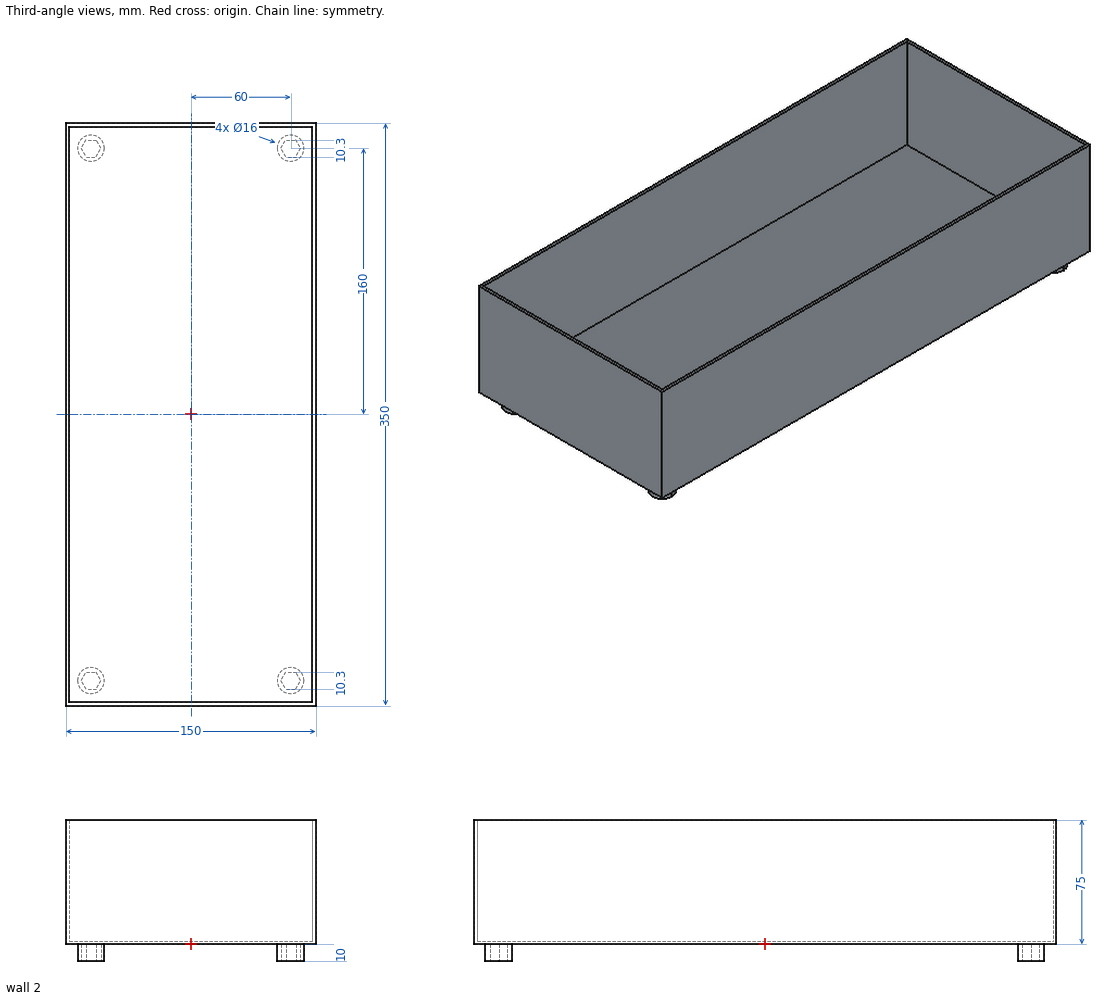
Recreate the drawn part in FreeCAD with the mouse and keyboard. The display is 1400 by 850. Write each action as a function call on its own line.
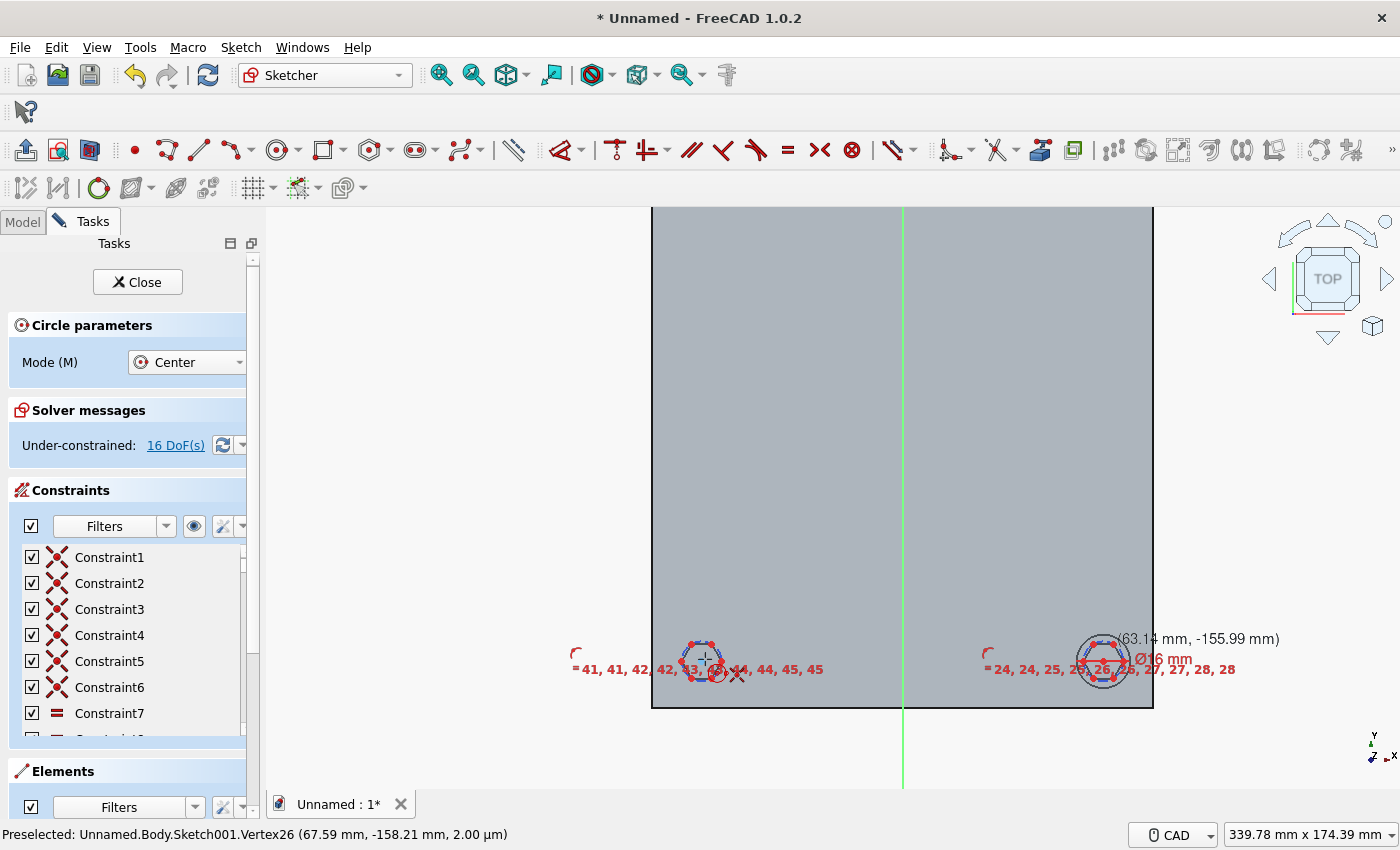
click(702, 661)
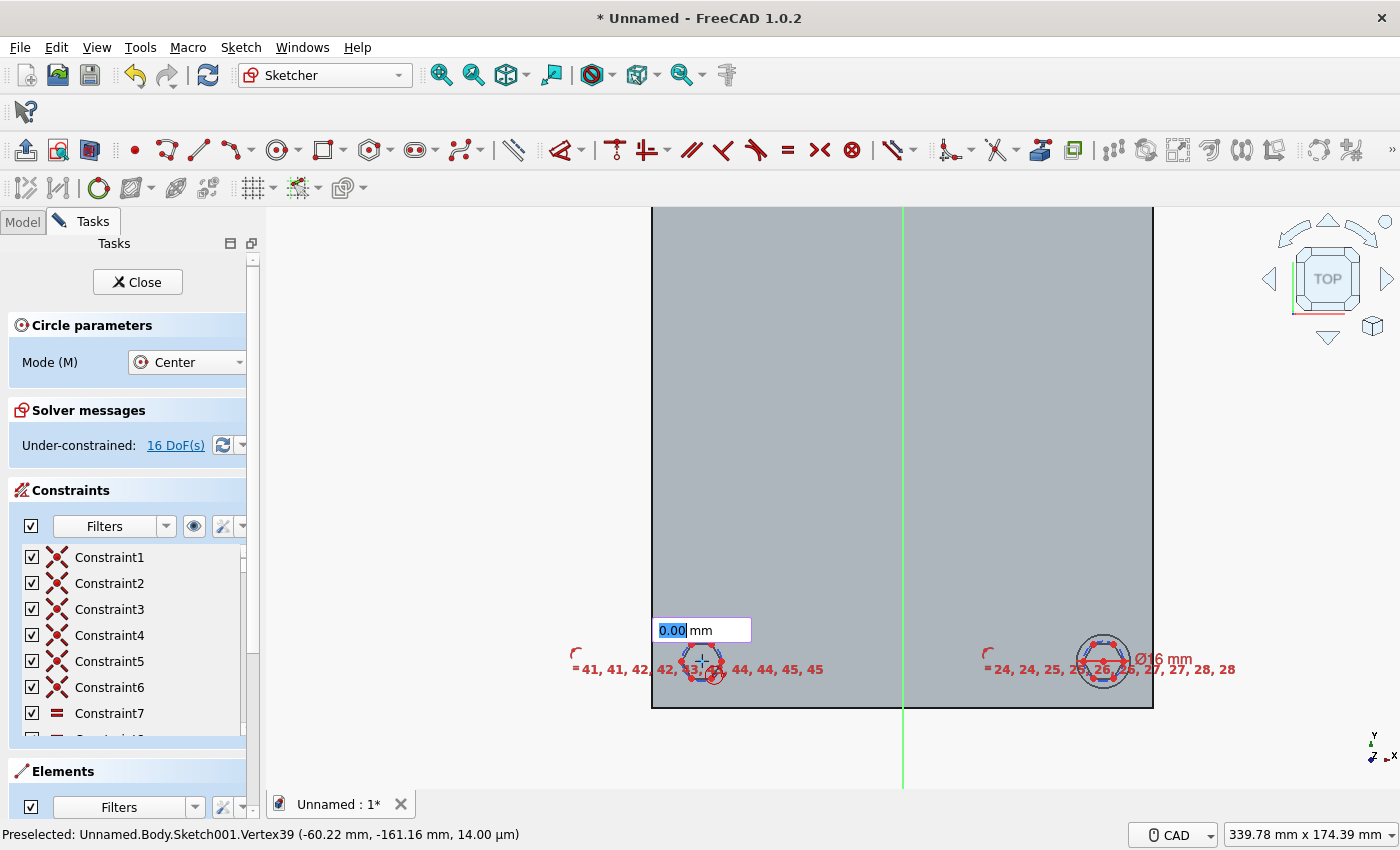
scroll(728, 648, up, 3)
move(727, 648)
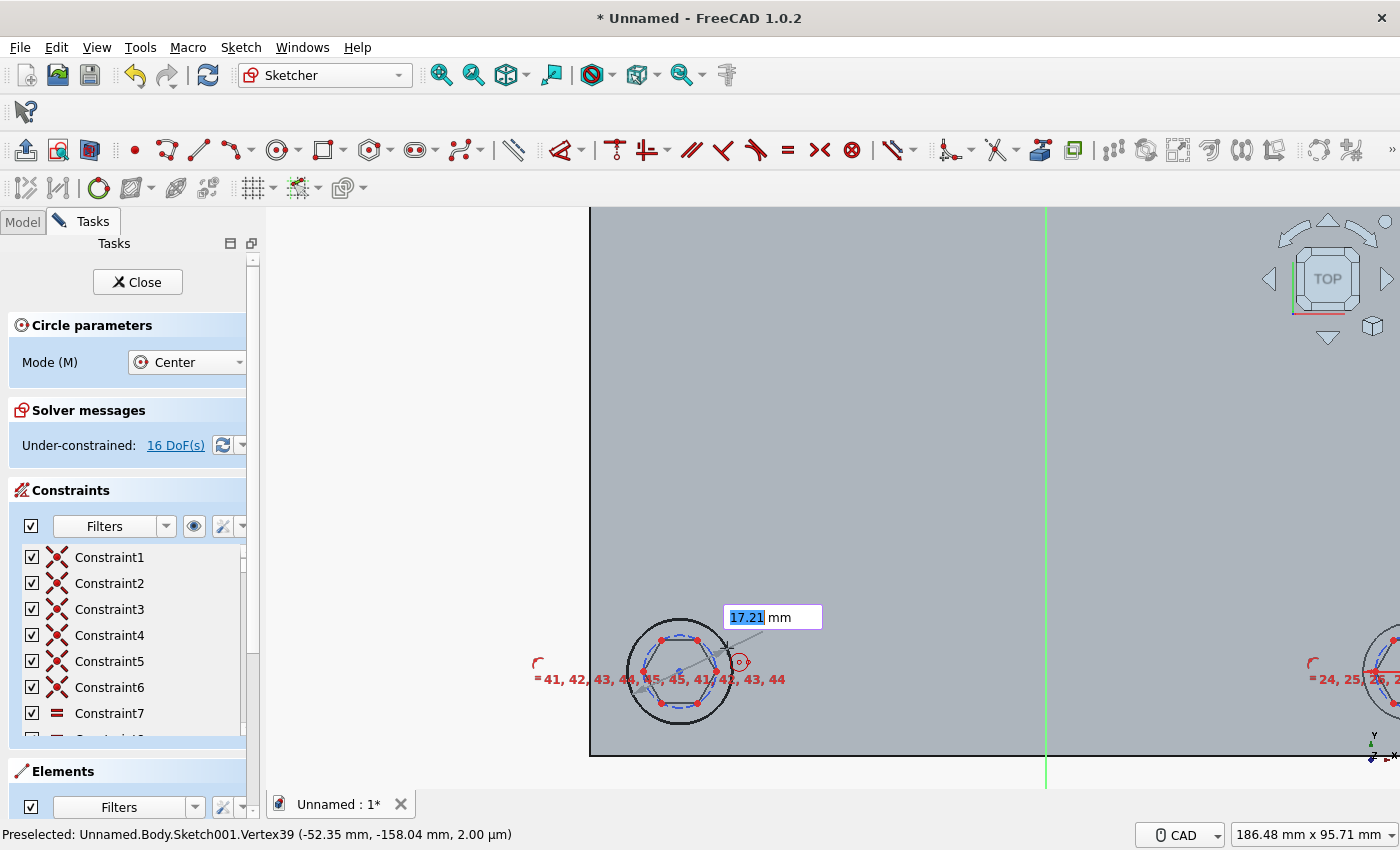
text(16)
key(Return)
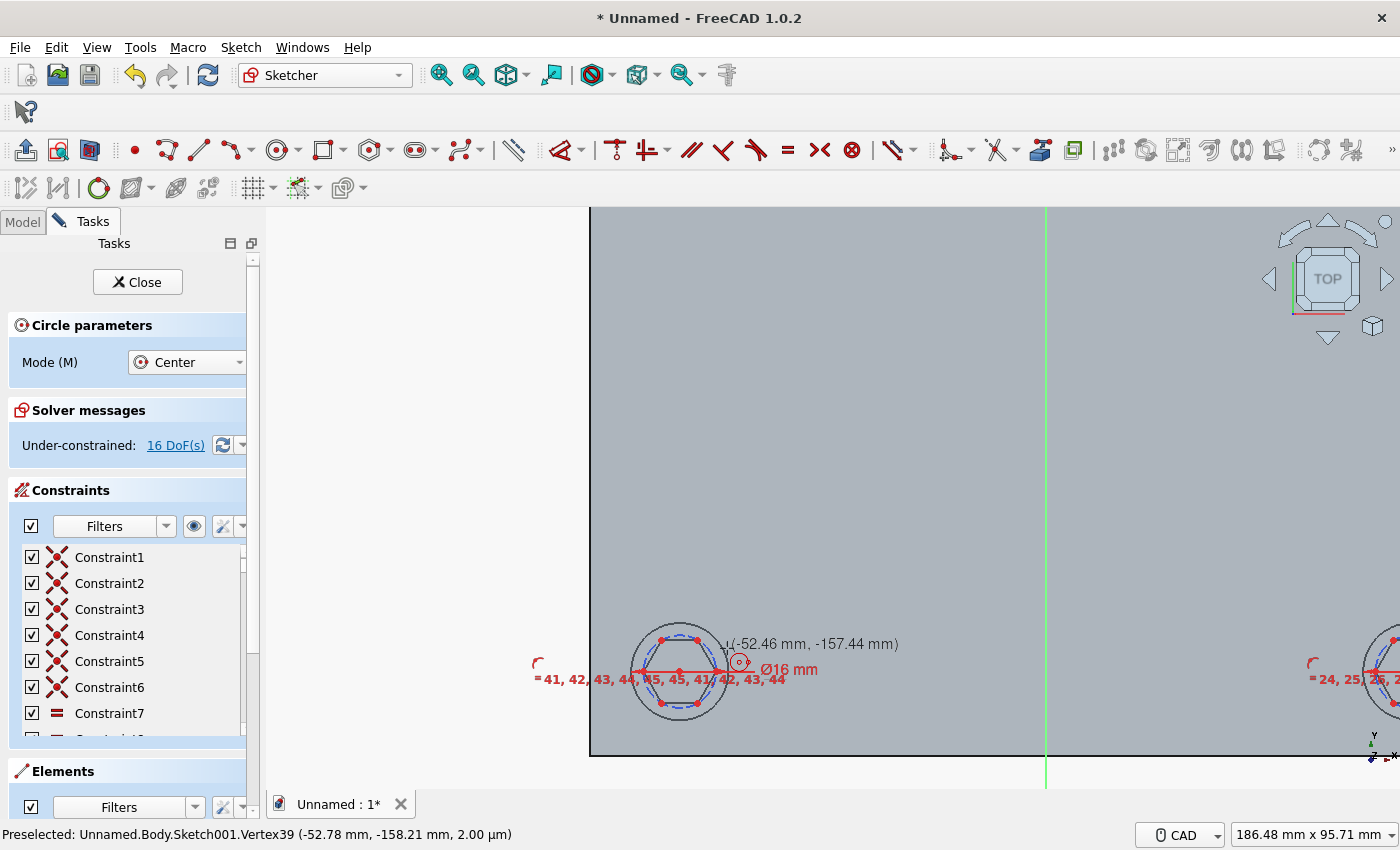
scroll(709, 658, down, 9)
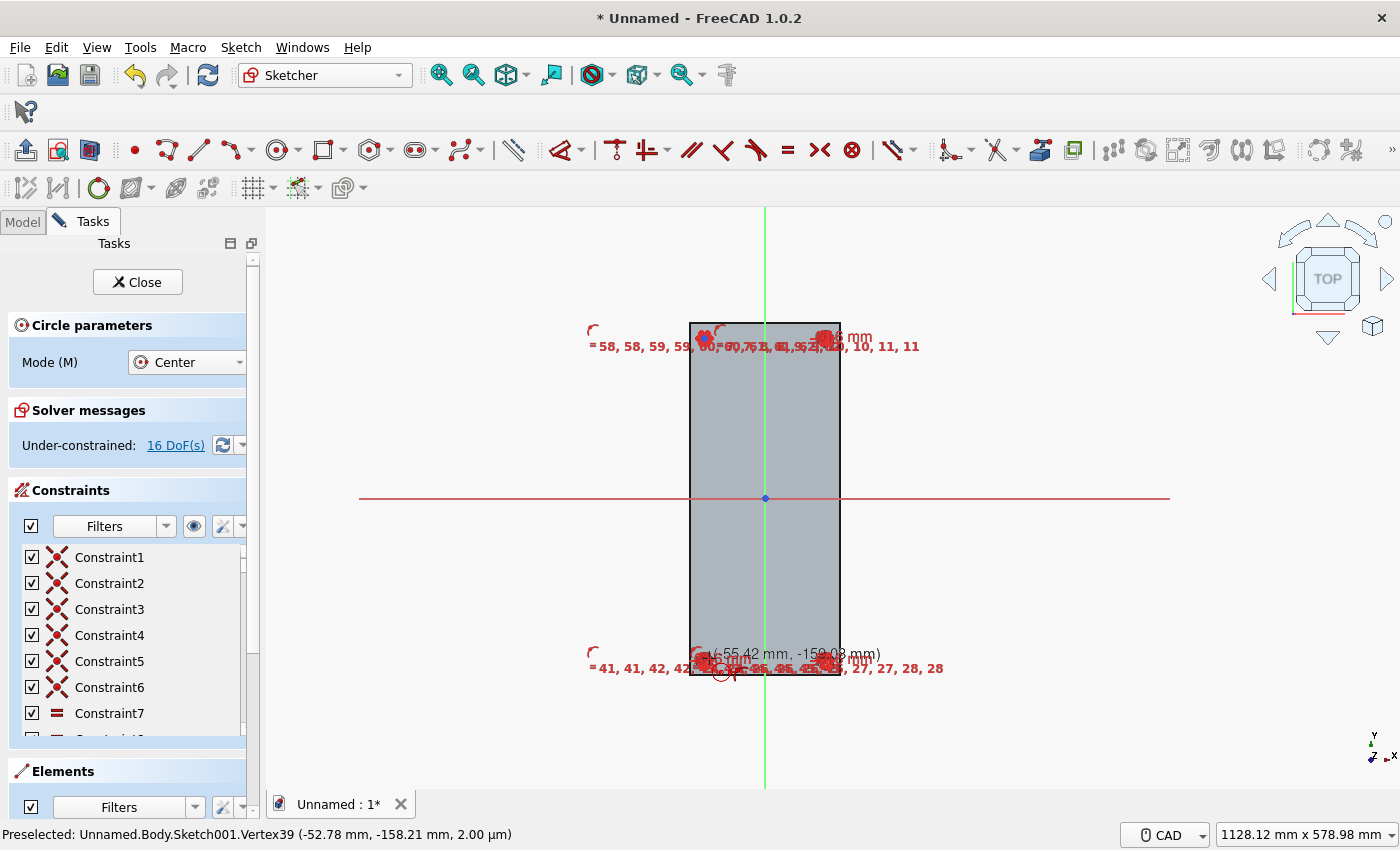
scroll(705, 338, up, 6)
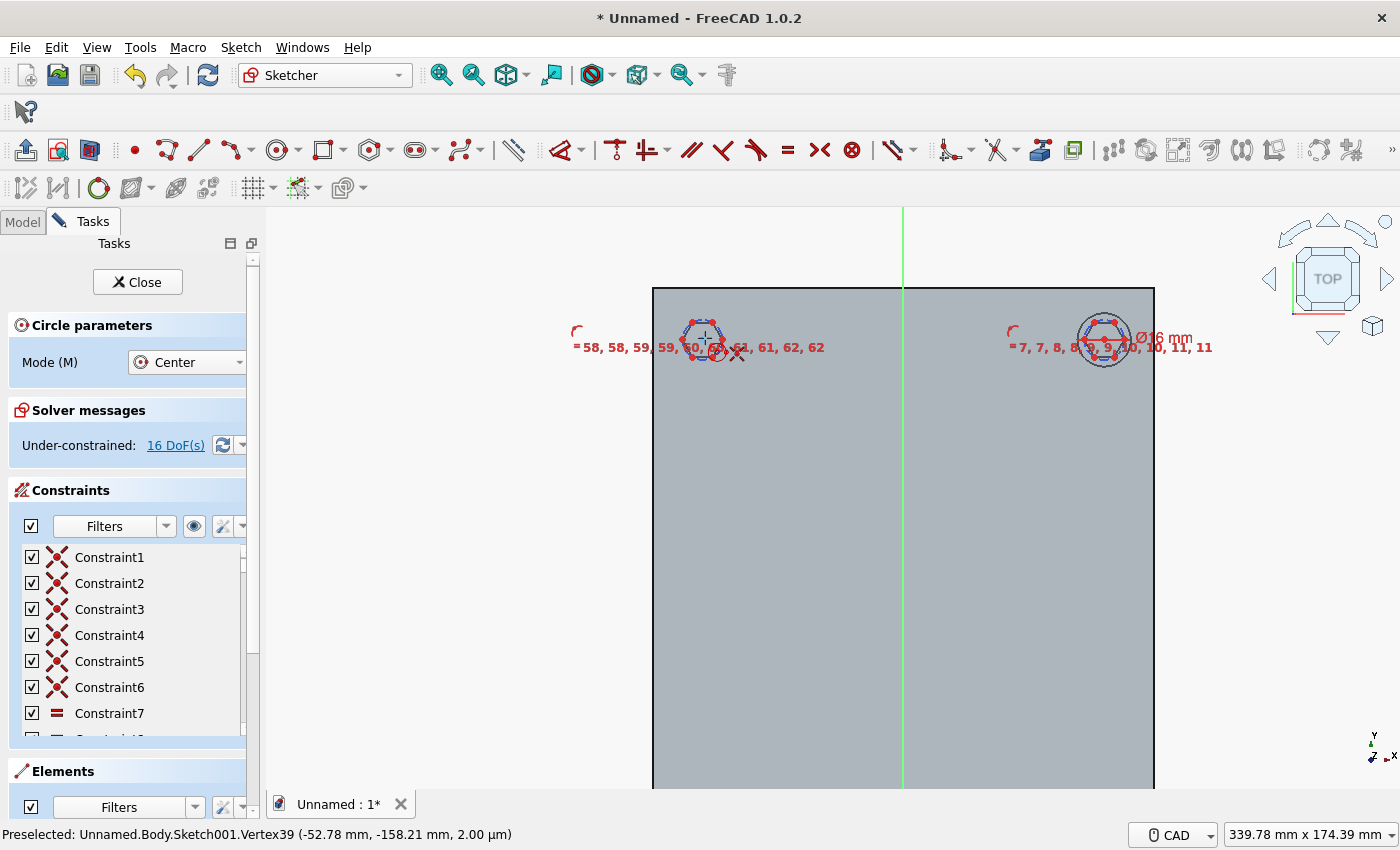
click(702, 340)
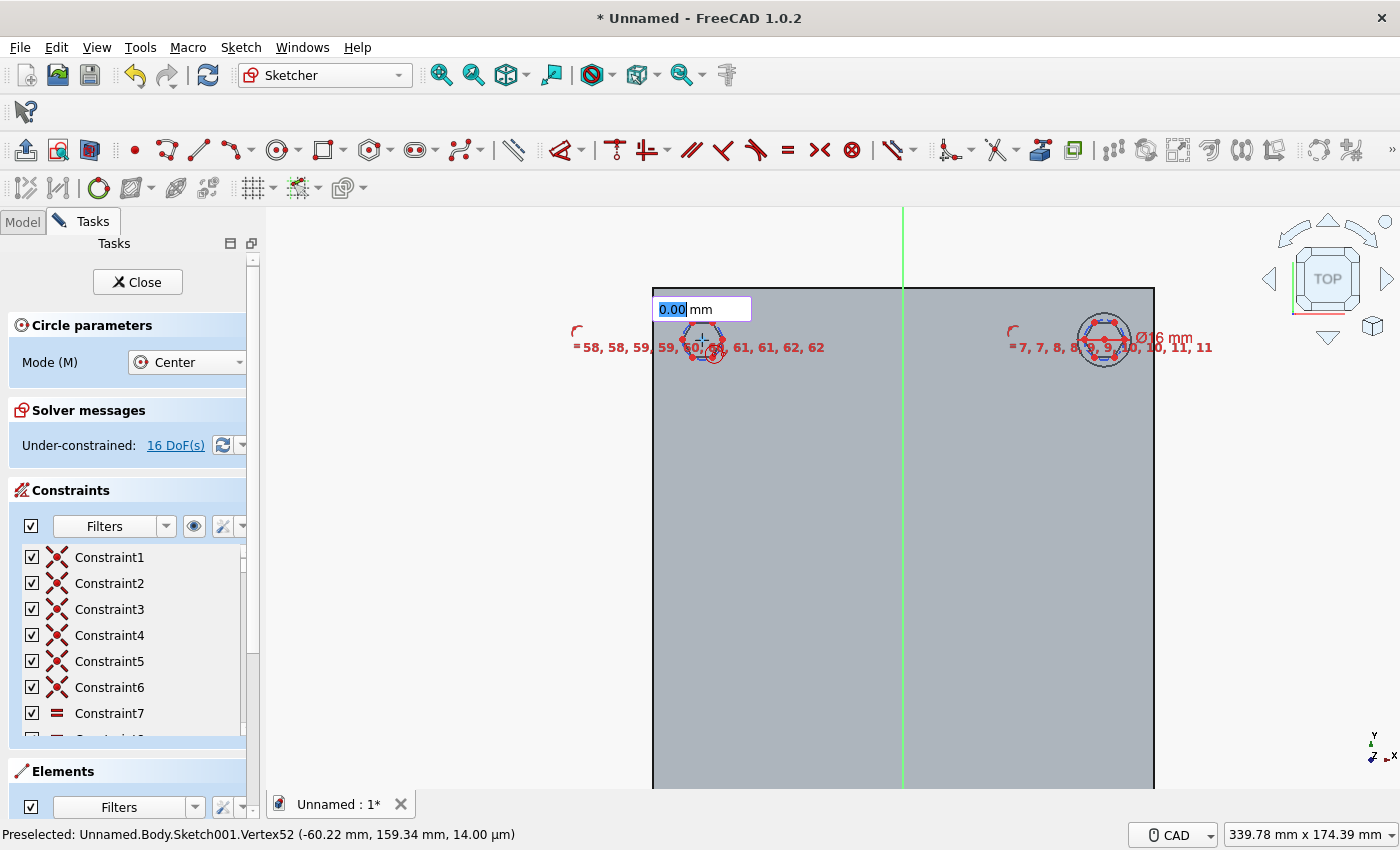
scroll(728, 329, up, 3)
move(728, 328)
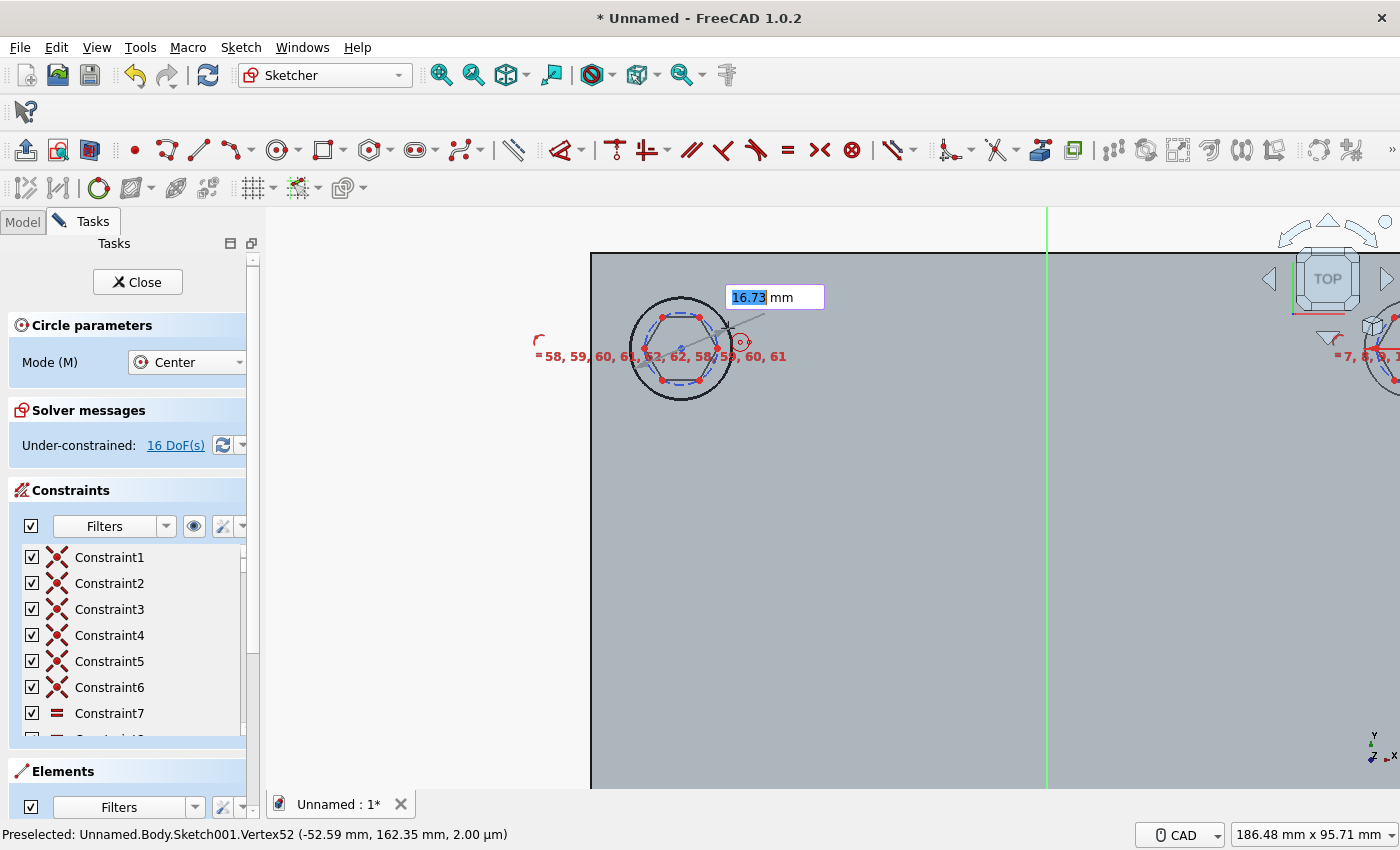
text(16)
key(Return)
key(Escape)